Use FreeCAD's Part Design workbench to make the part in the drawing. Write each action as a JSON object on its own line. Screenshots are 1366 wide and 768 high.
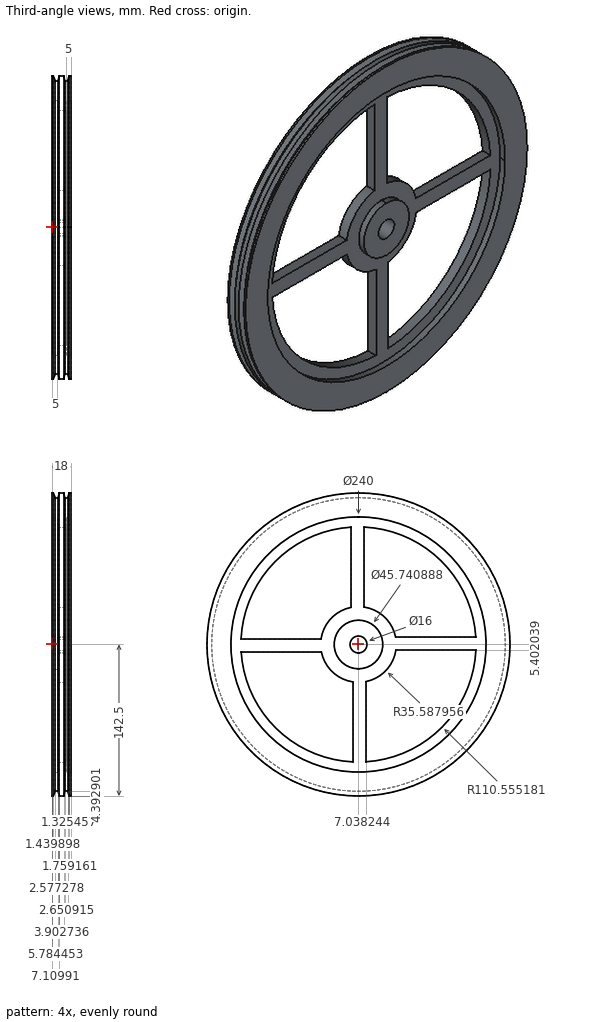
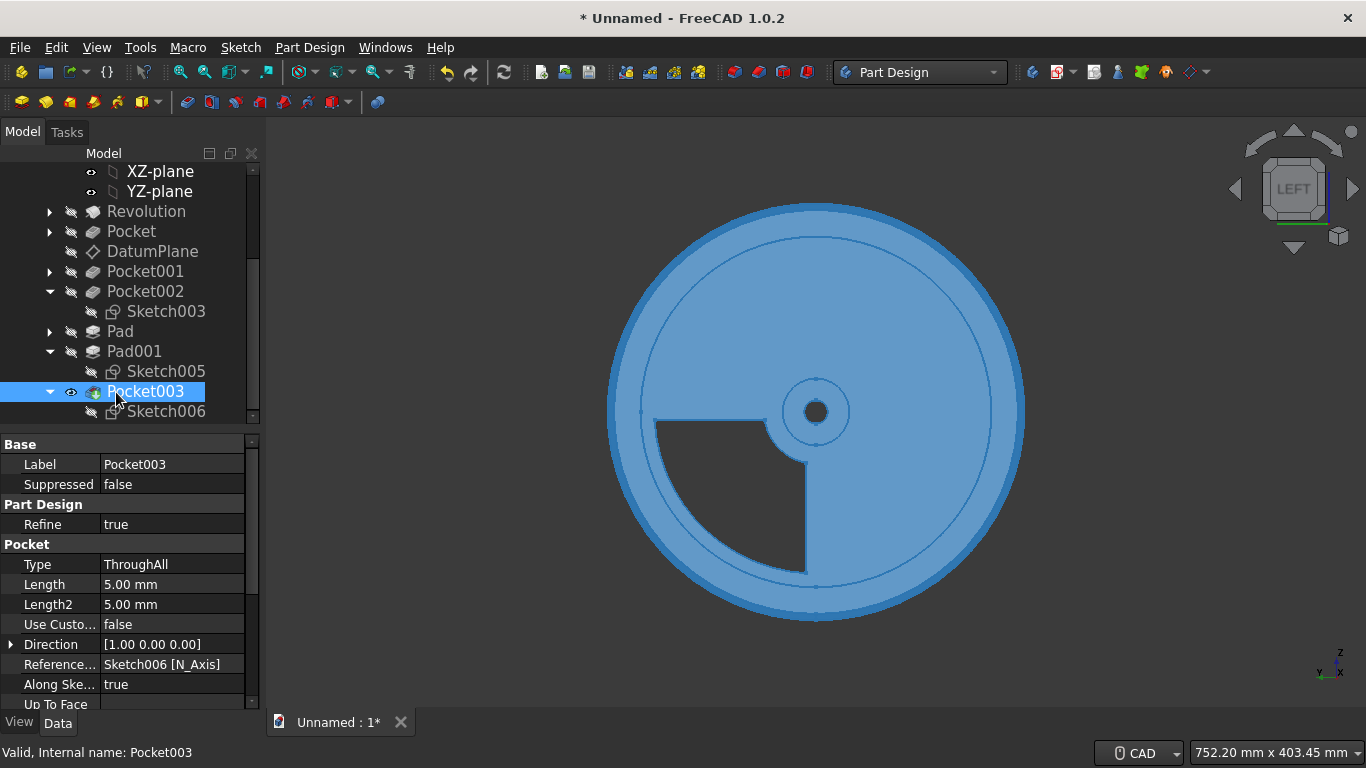
{"action": "left_click", "coordinate": [674, 72]}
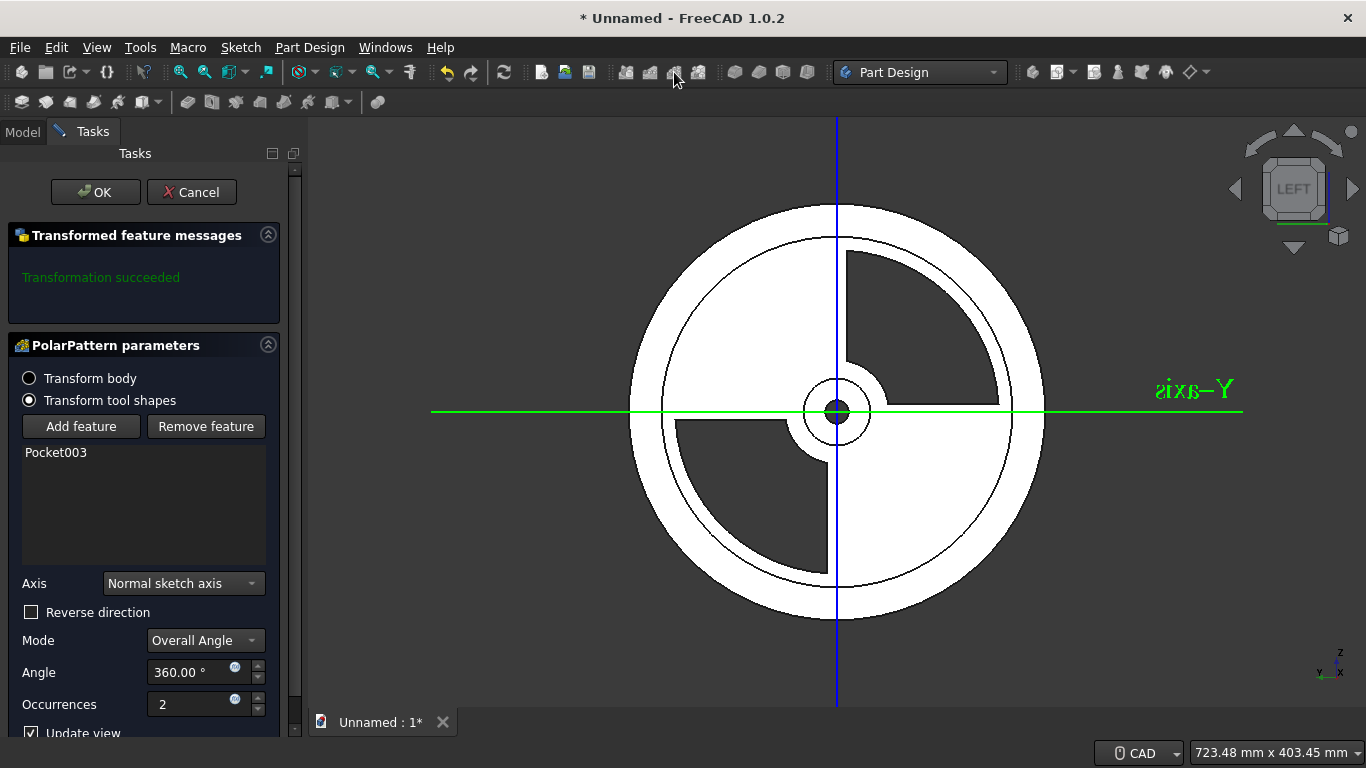
{"action": "left_click", "coordinate": [184, 584]}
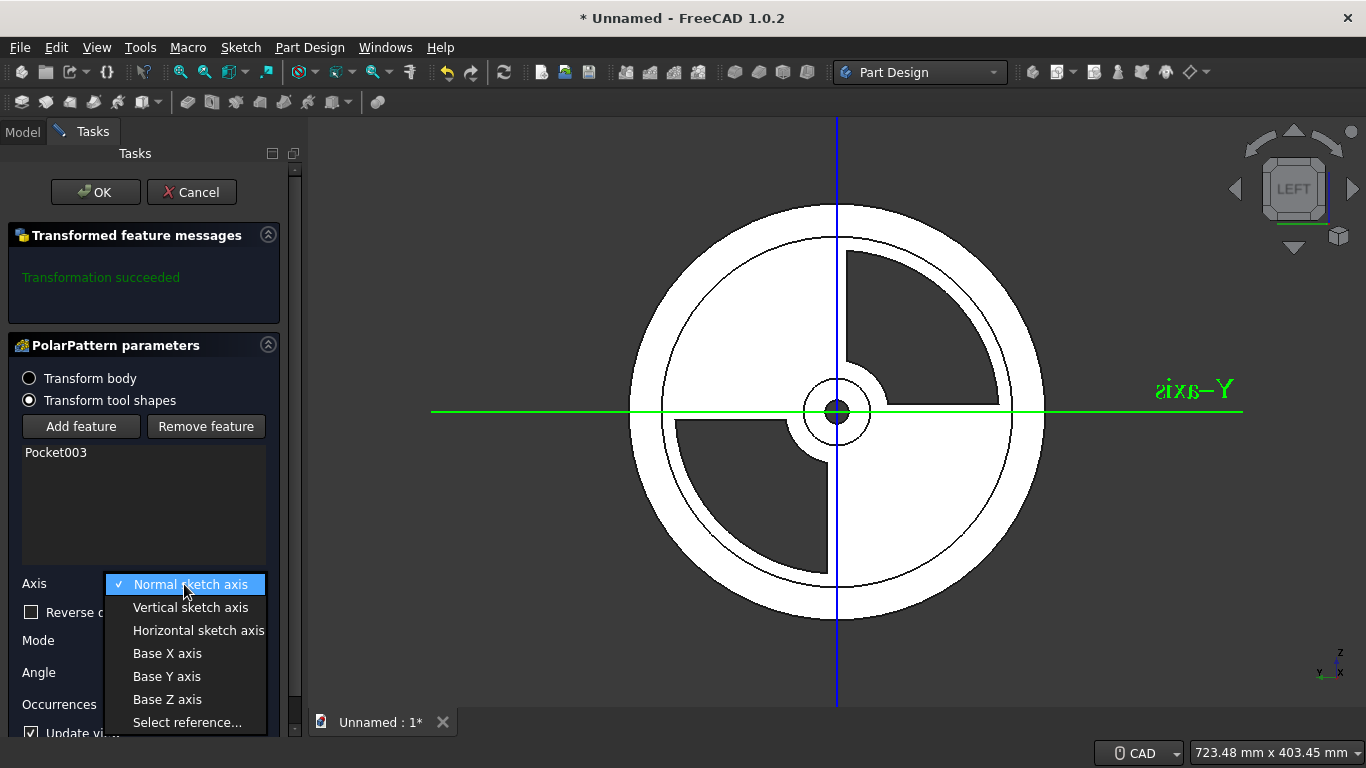
{"action": "left_click", "coordinate": [184, 654]}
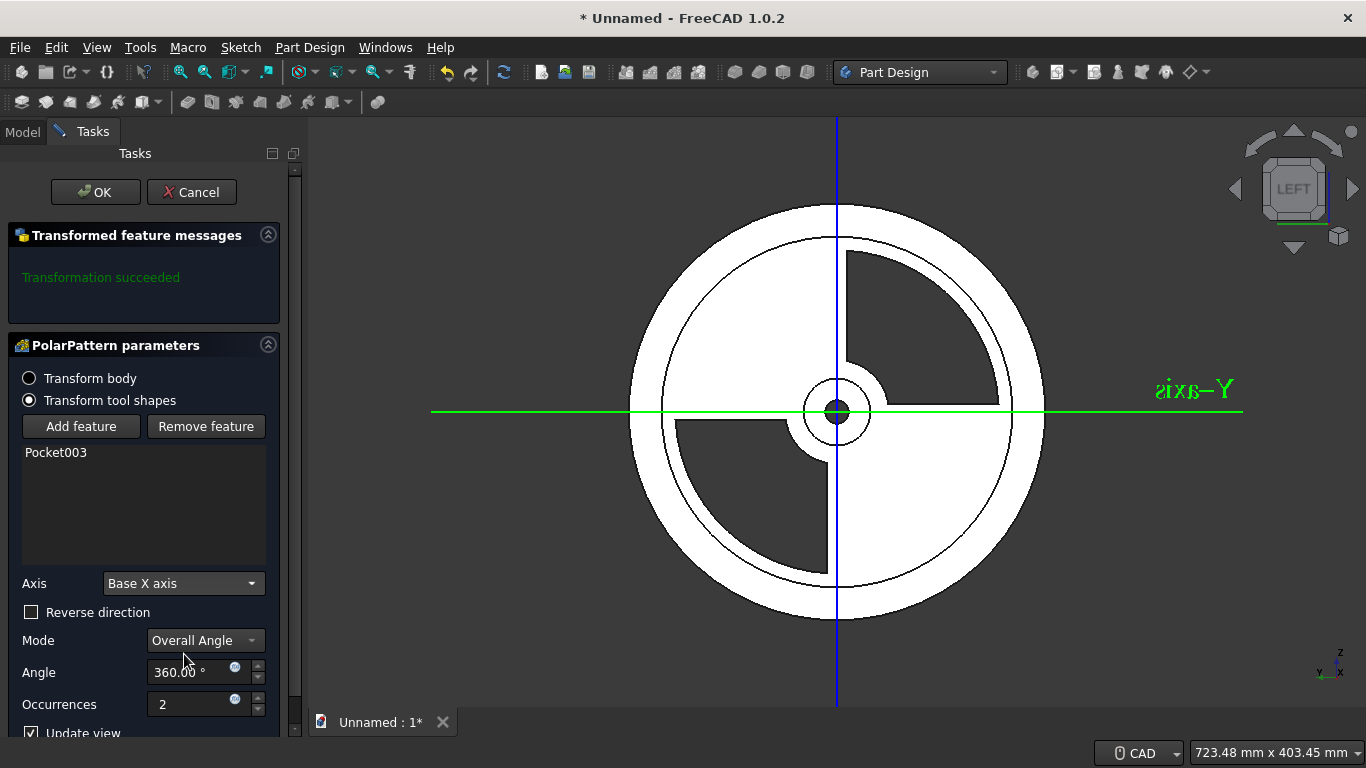
{"action": "triple_click", "coordinate": [198, 704]}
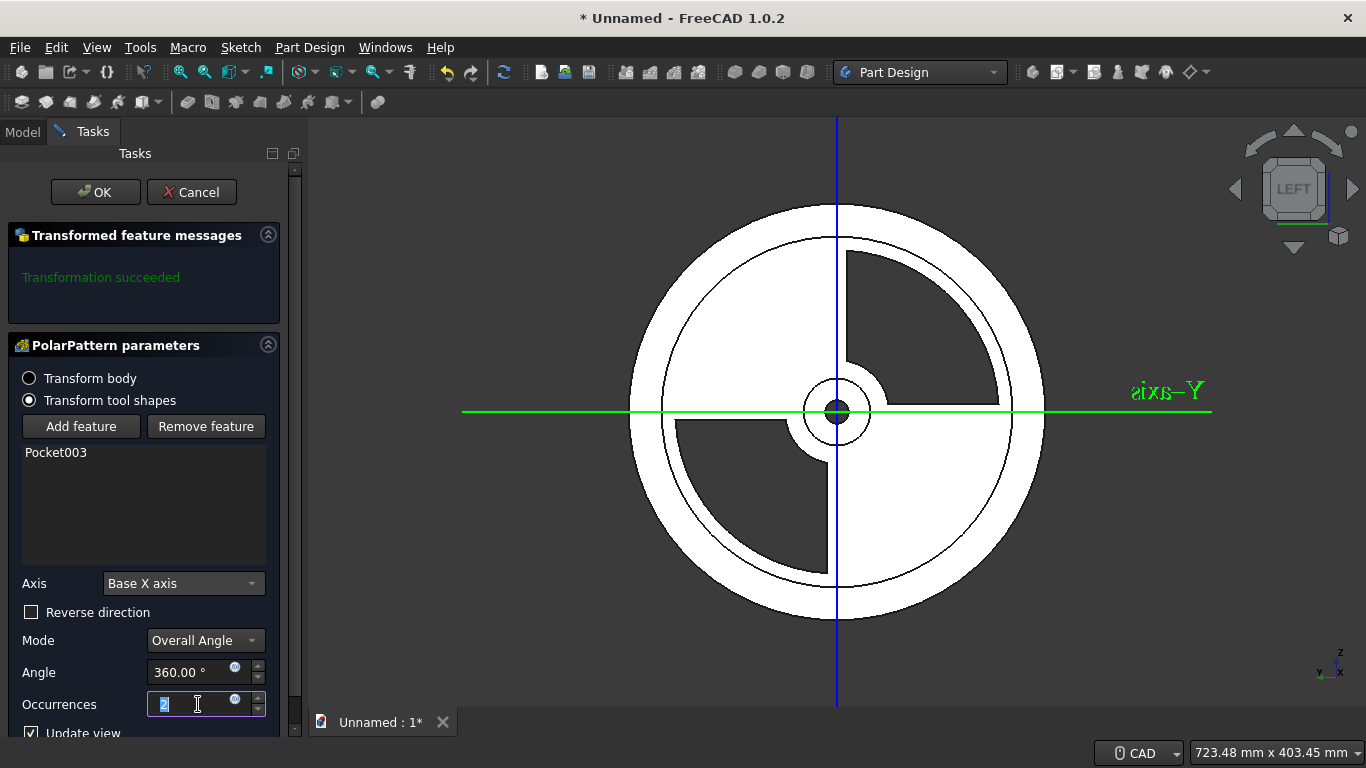
{"action": "type", "text": "4"}
{"action": "key", "text": "Tab"}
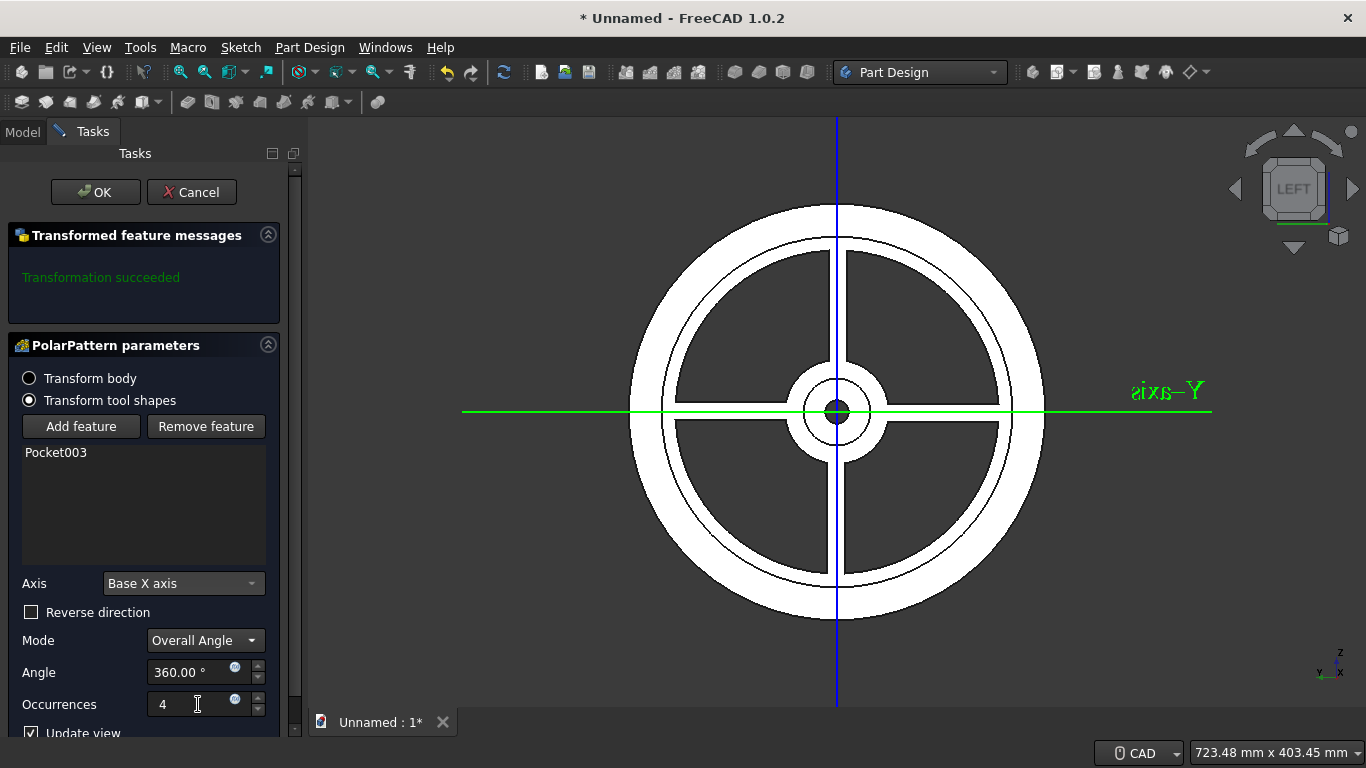
{"action": "left_click", "coordinate": [96, 192]}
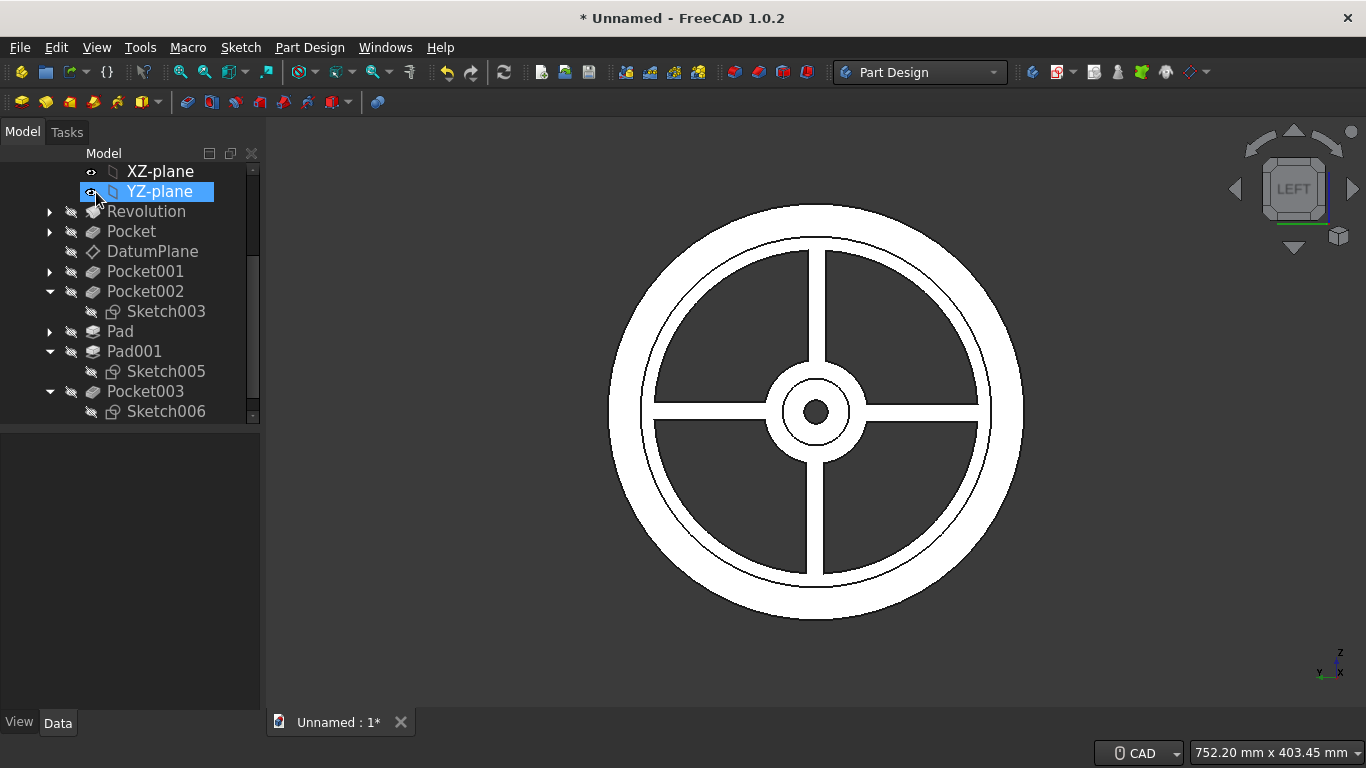
{"action": "key", "text": "0"}